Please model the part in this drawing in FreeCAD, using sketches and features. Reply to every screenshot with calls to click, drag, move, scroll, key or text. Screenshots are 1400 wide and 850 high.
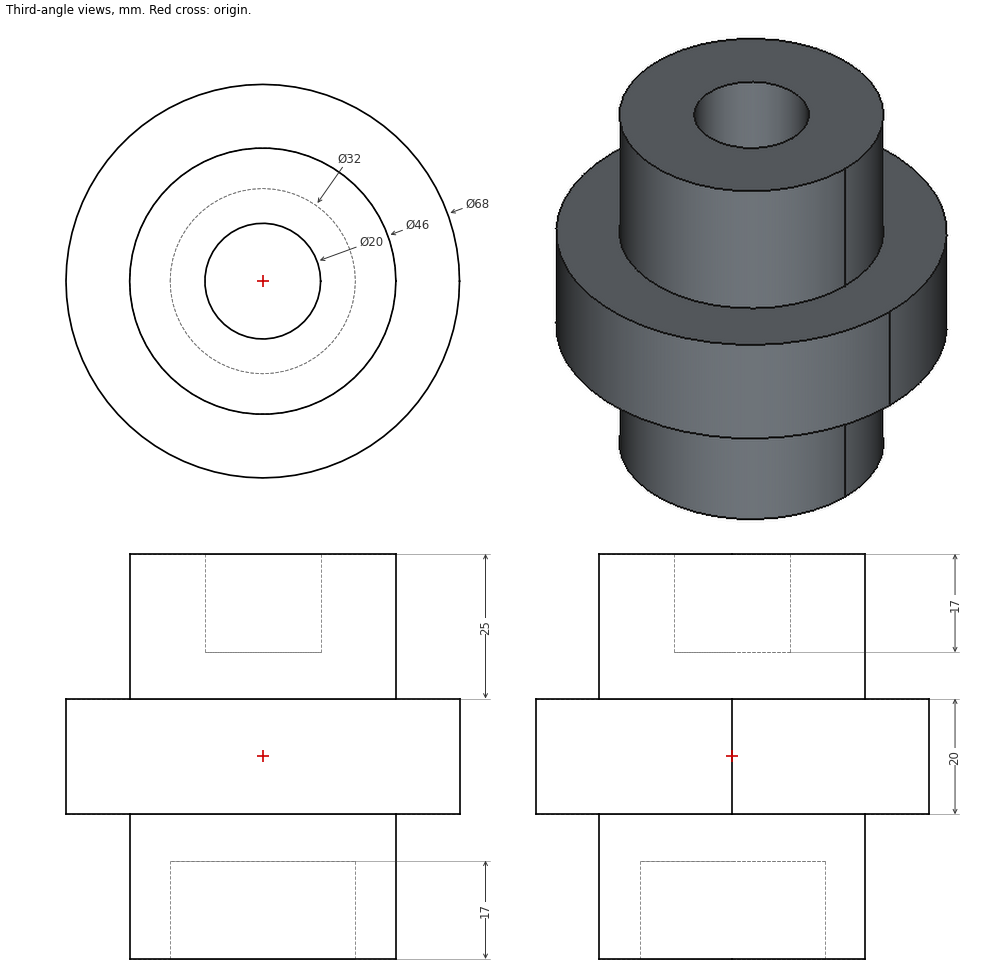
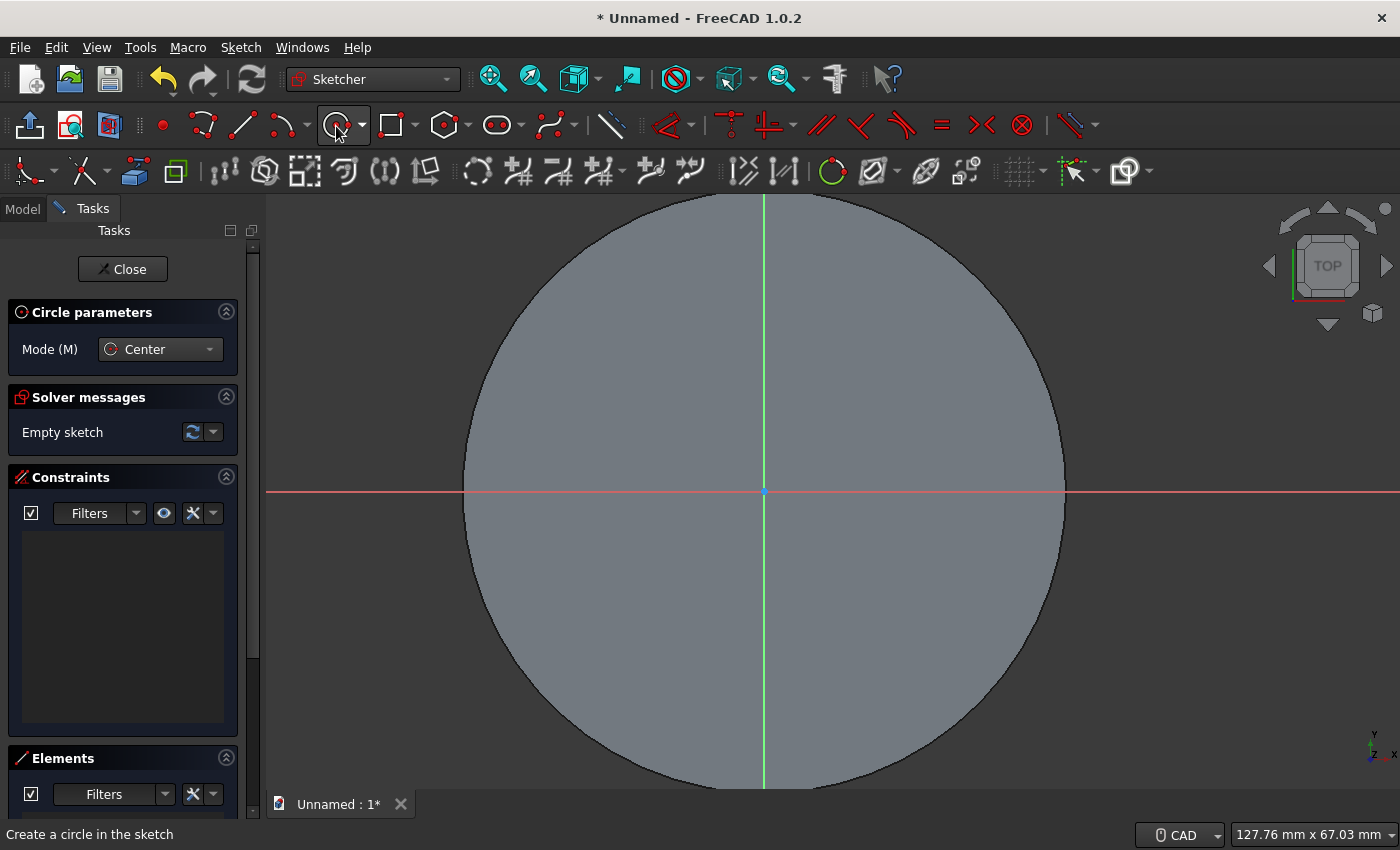
click(764, 492)
move(909, 347)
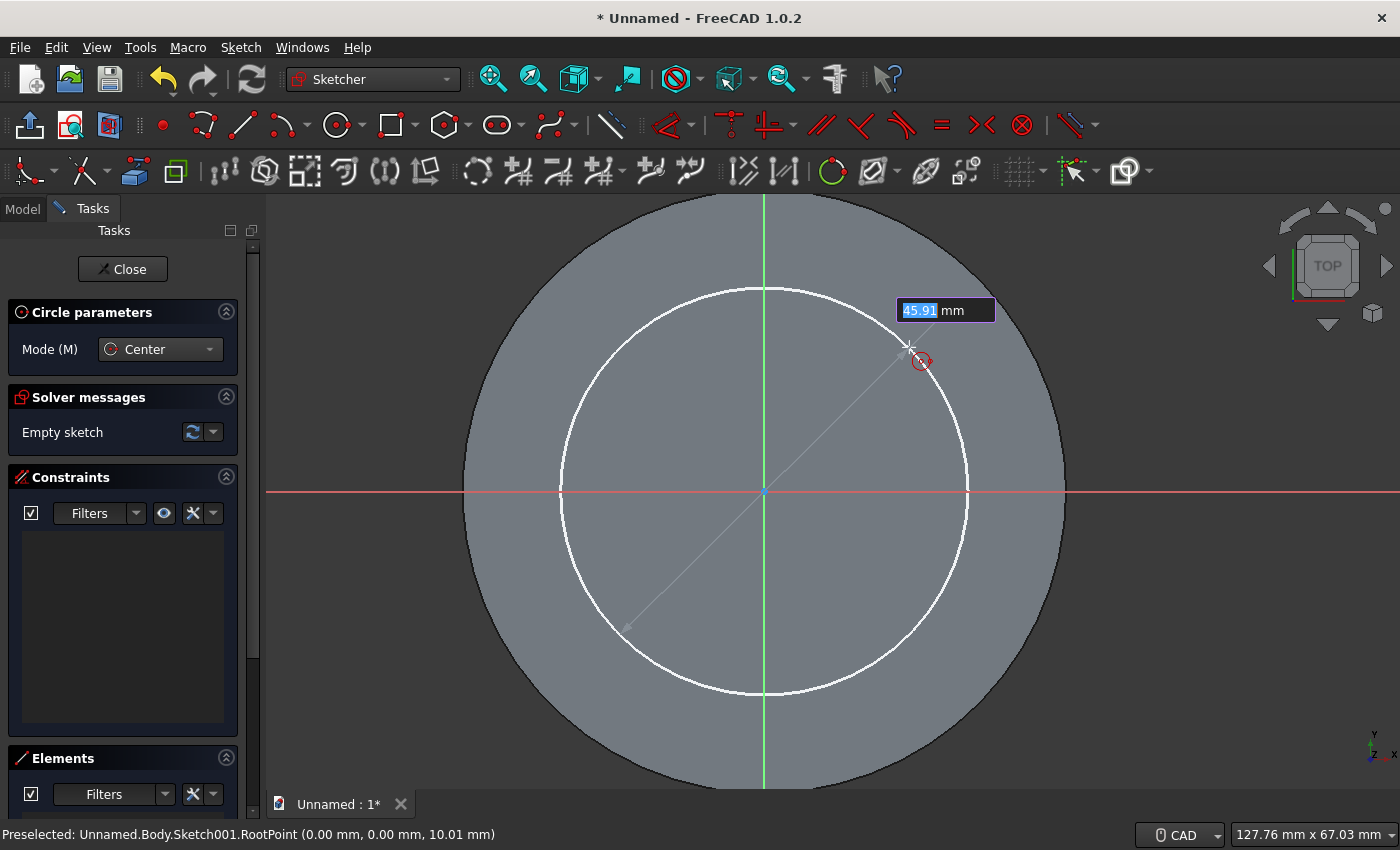
text(46)
key(Return)
key(Escape)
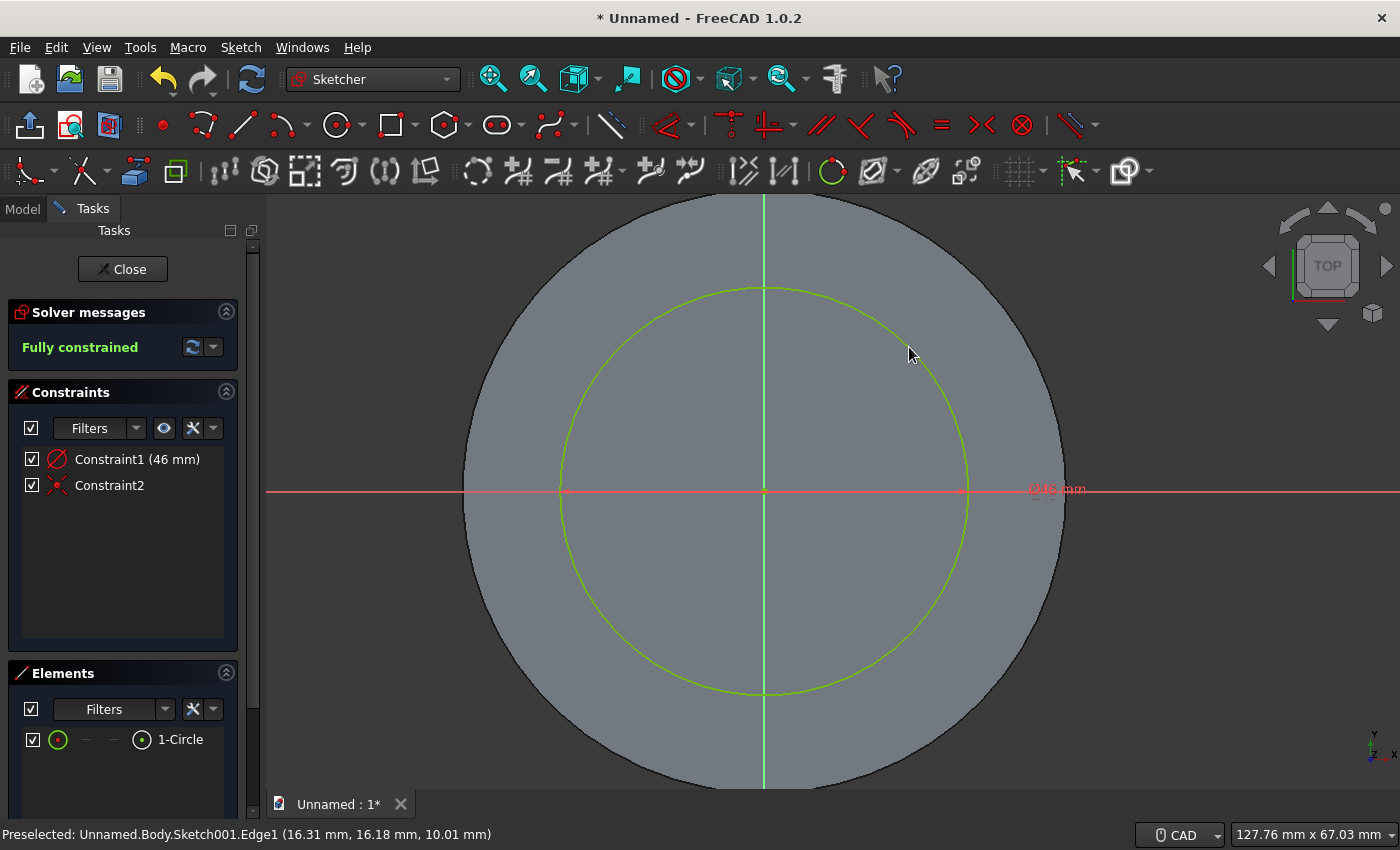
click(123, 269)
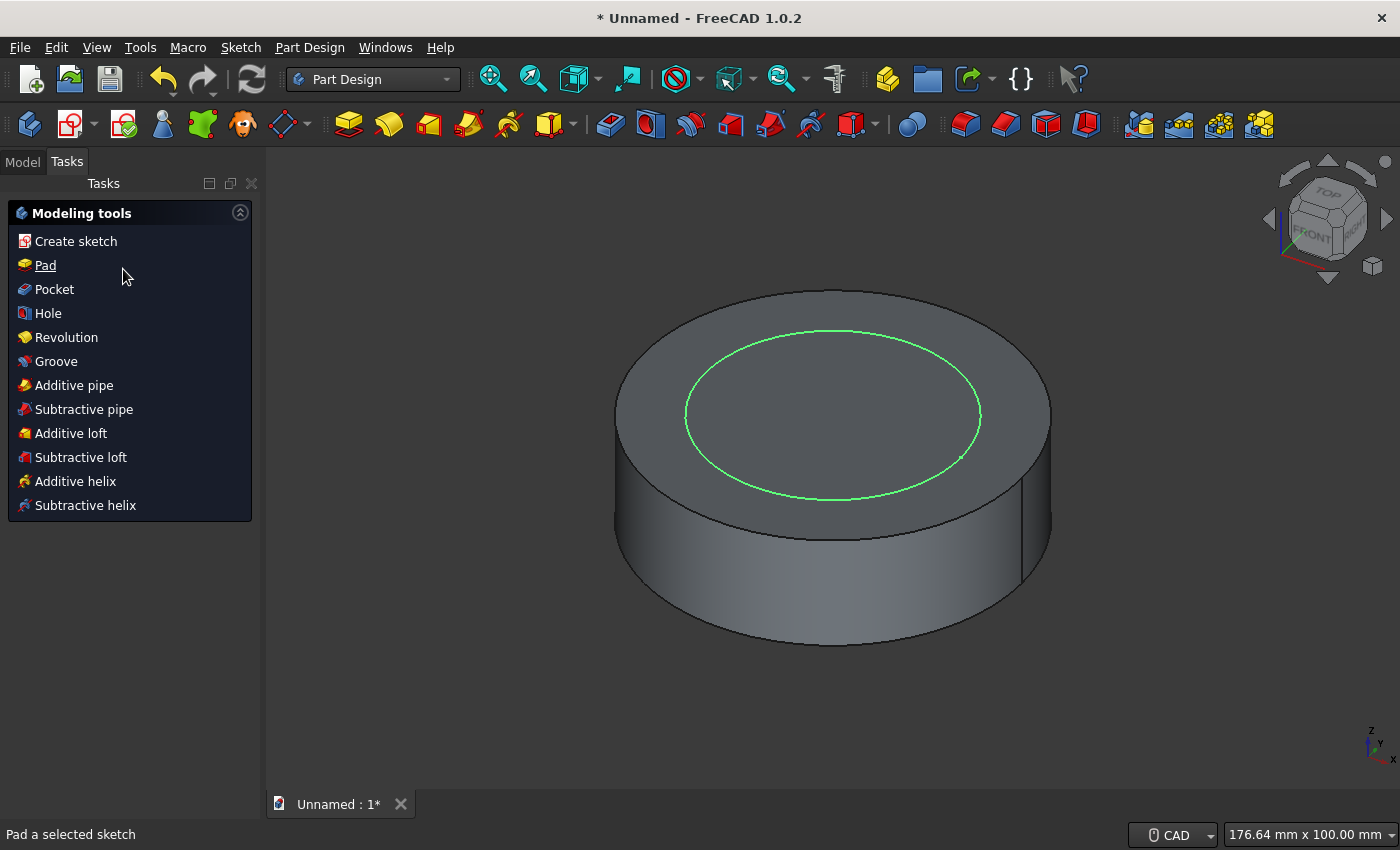
click(350, 124)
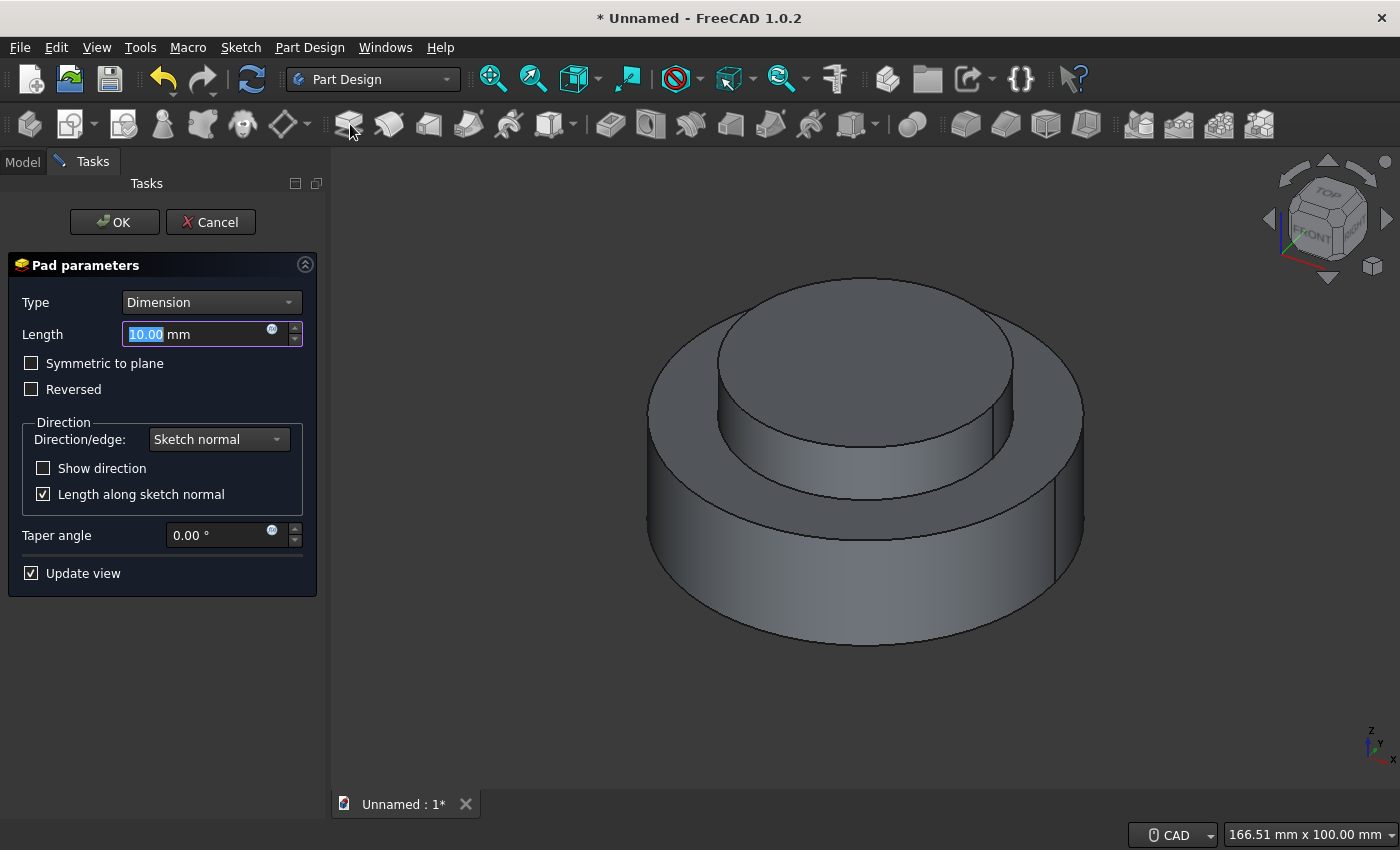
text(25)
key(Tab)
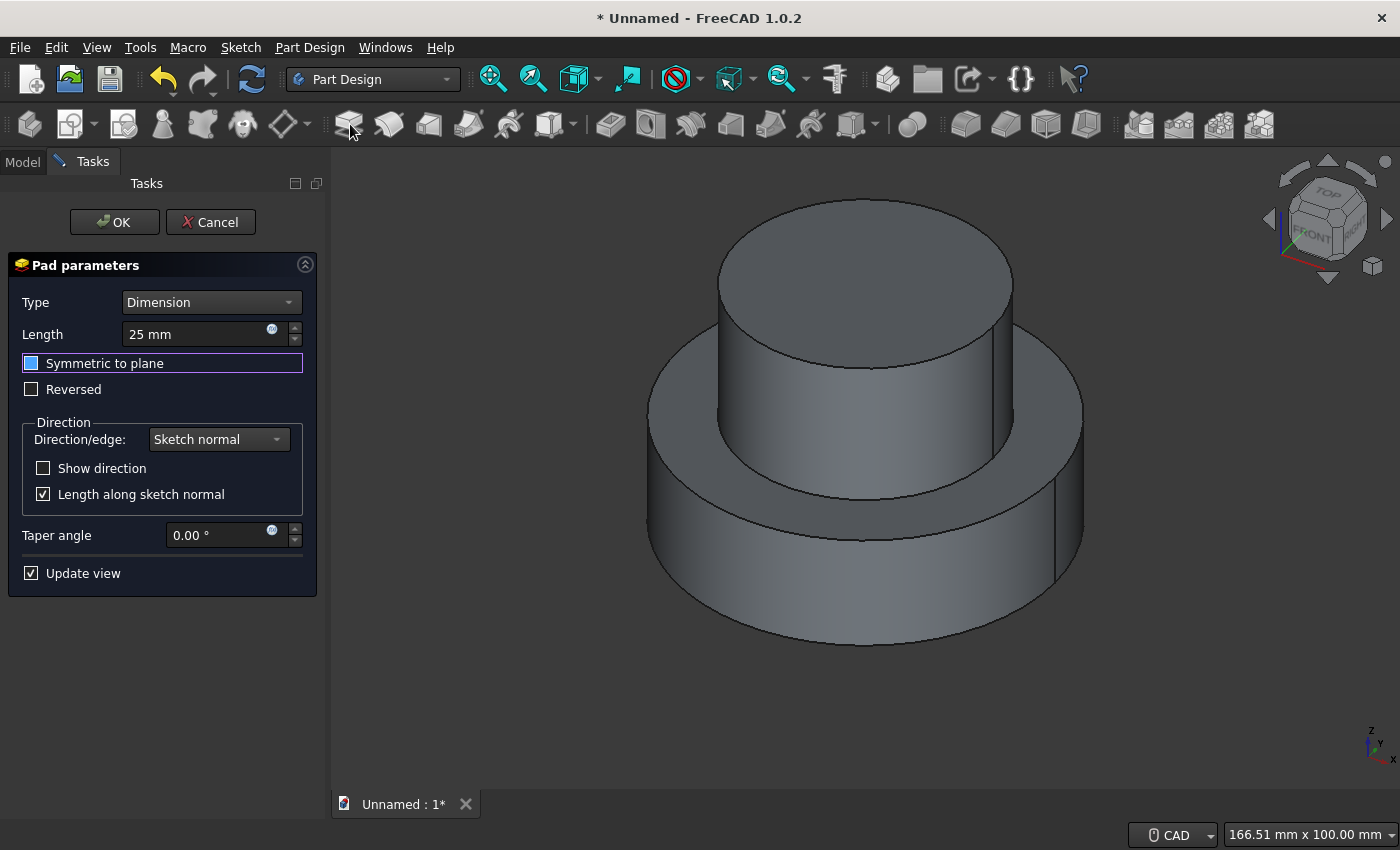
click(115, 222)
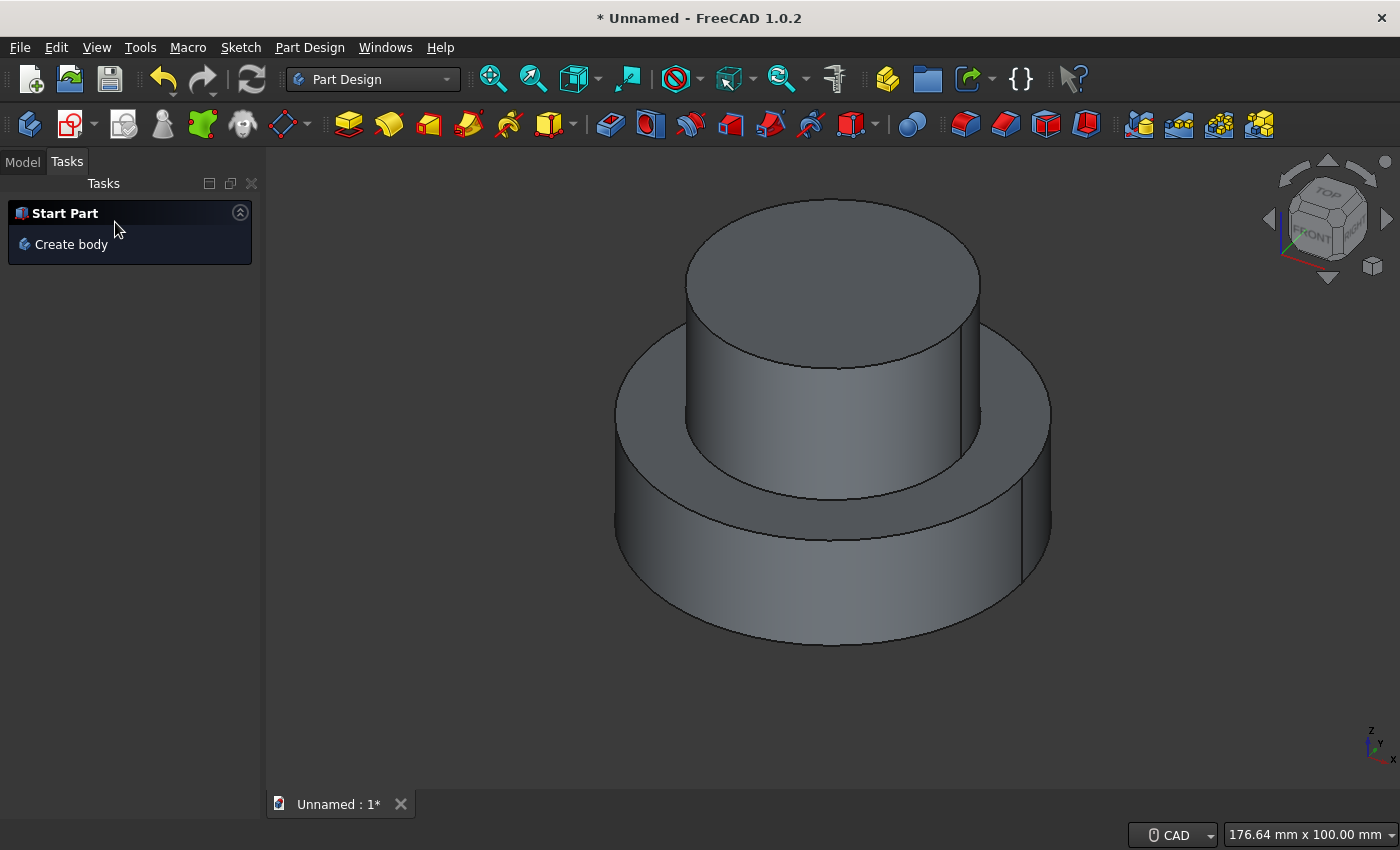
click(494, 80)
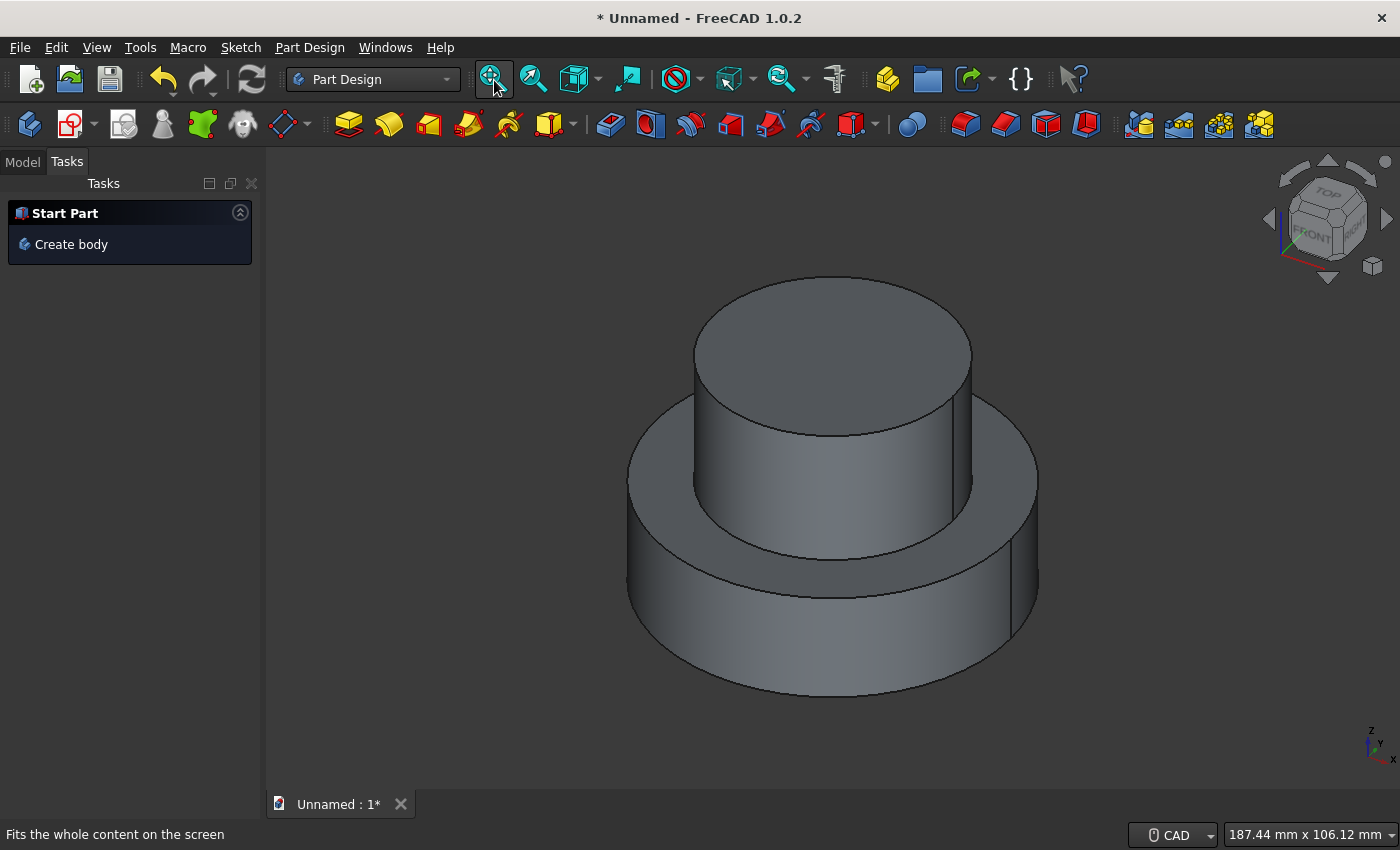
click(23, 161)